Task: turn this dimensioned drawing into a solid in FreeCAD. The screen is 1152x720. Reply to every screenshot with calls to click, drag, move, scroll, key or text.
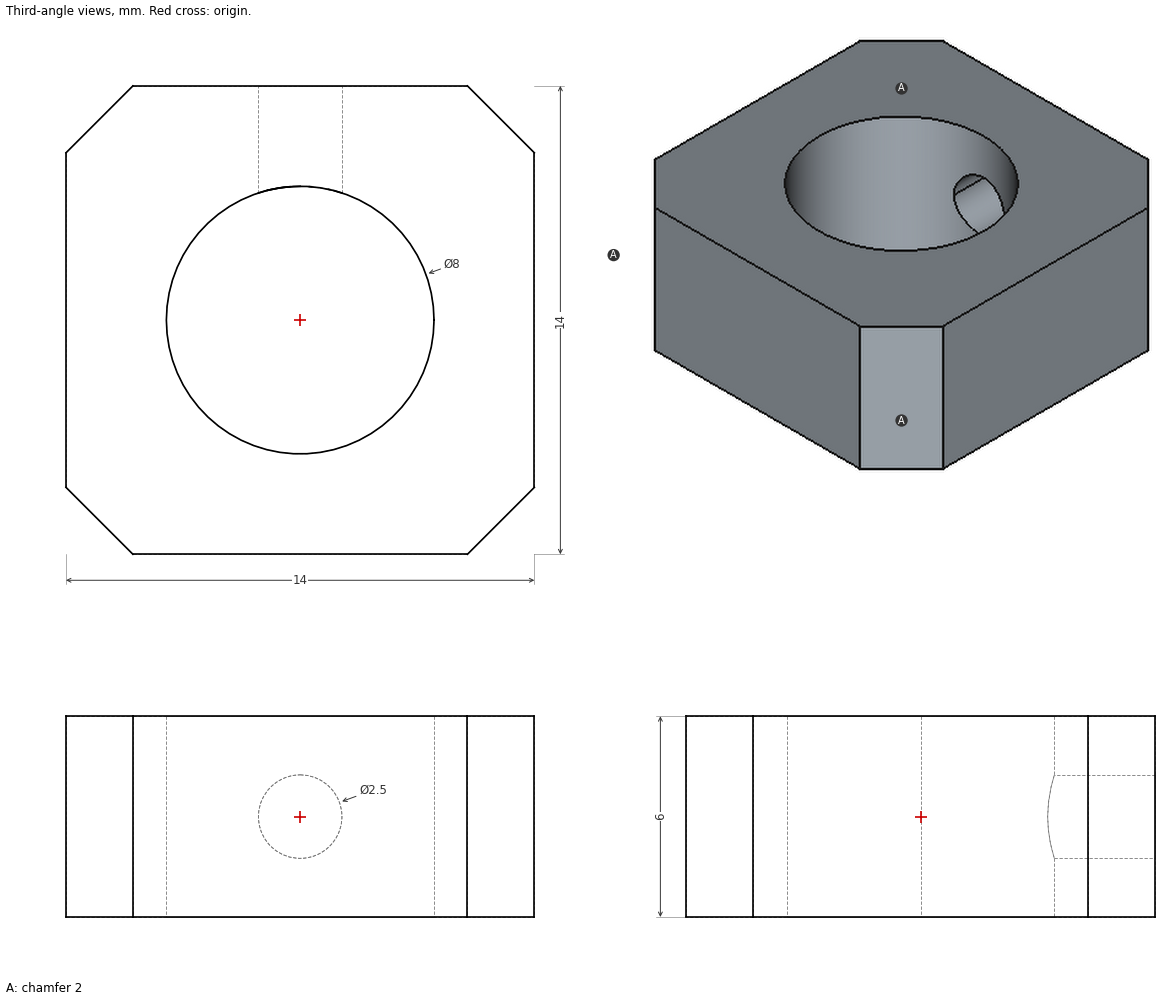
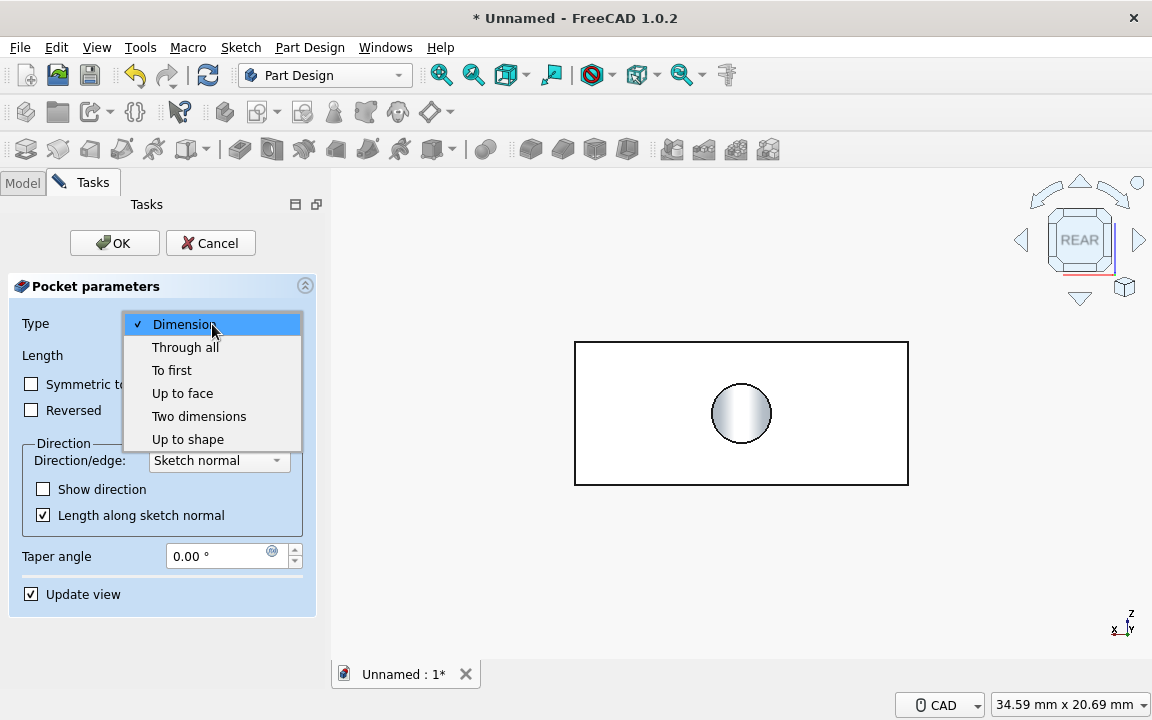
click(212, 370)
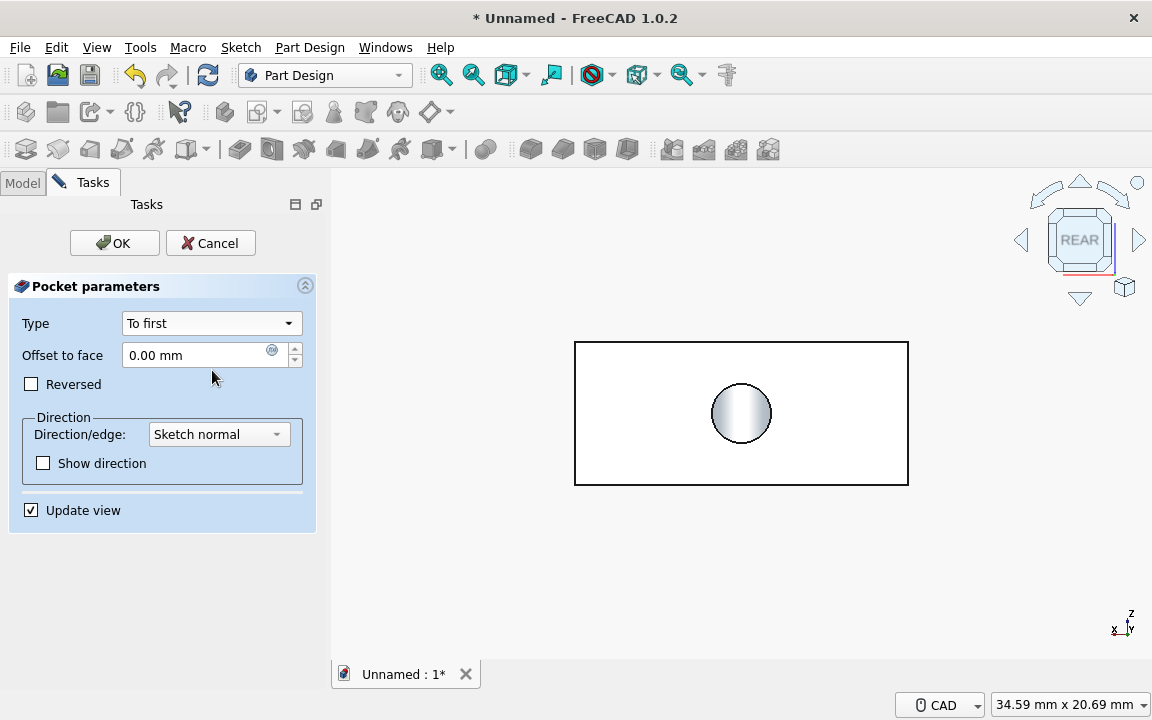
click(115, 243)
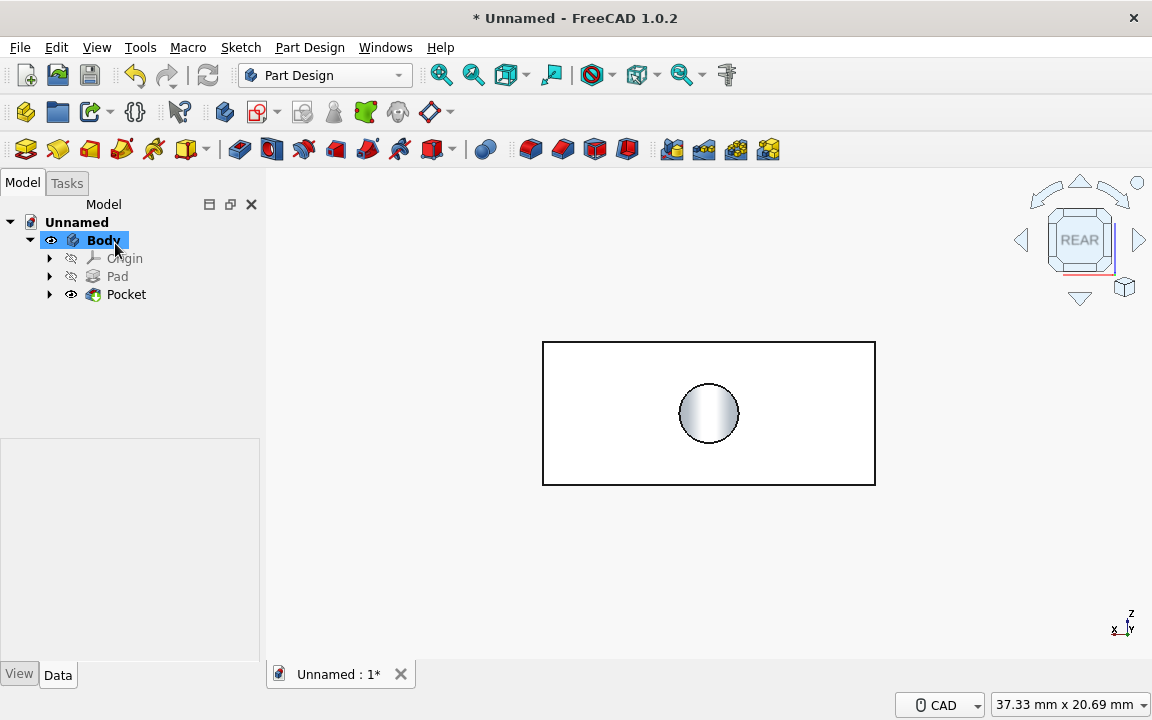
click(442, 76)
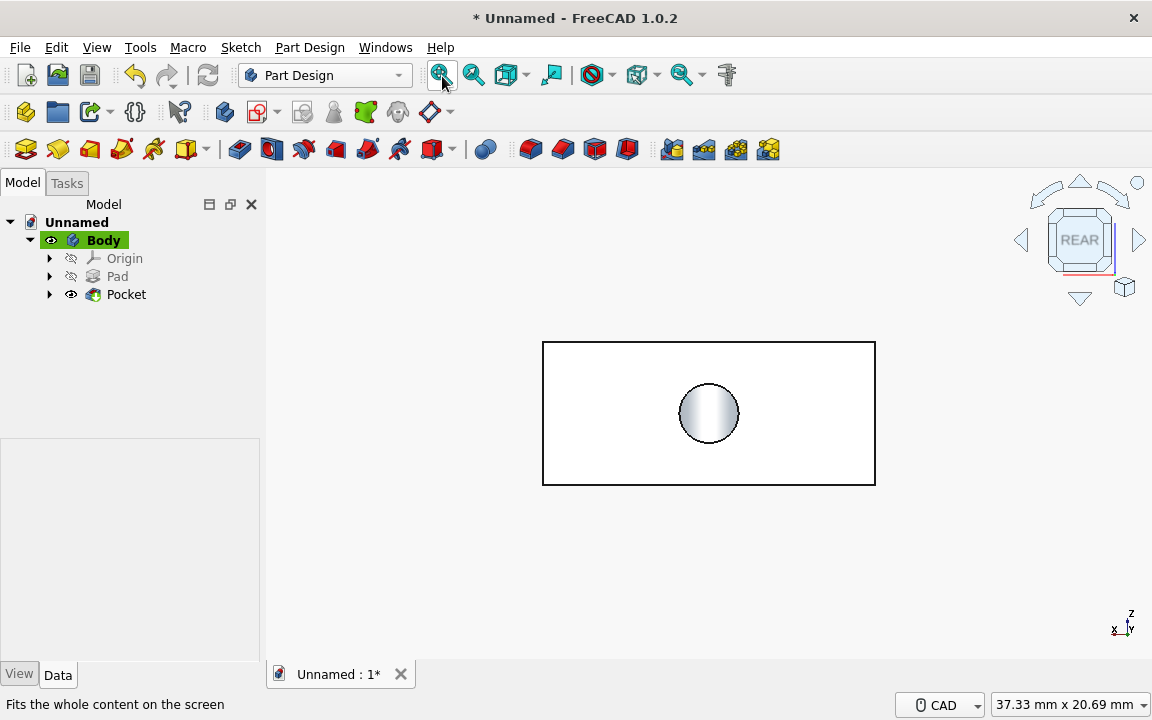
click(875, 412)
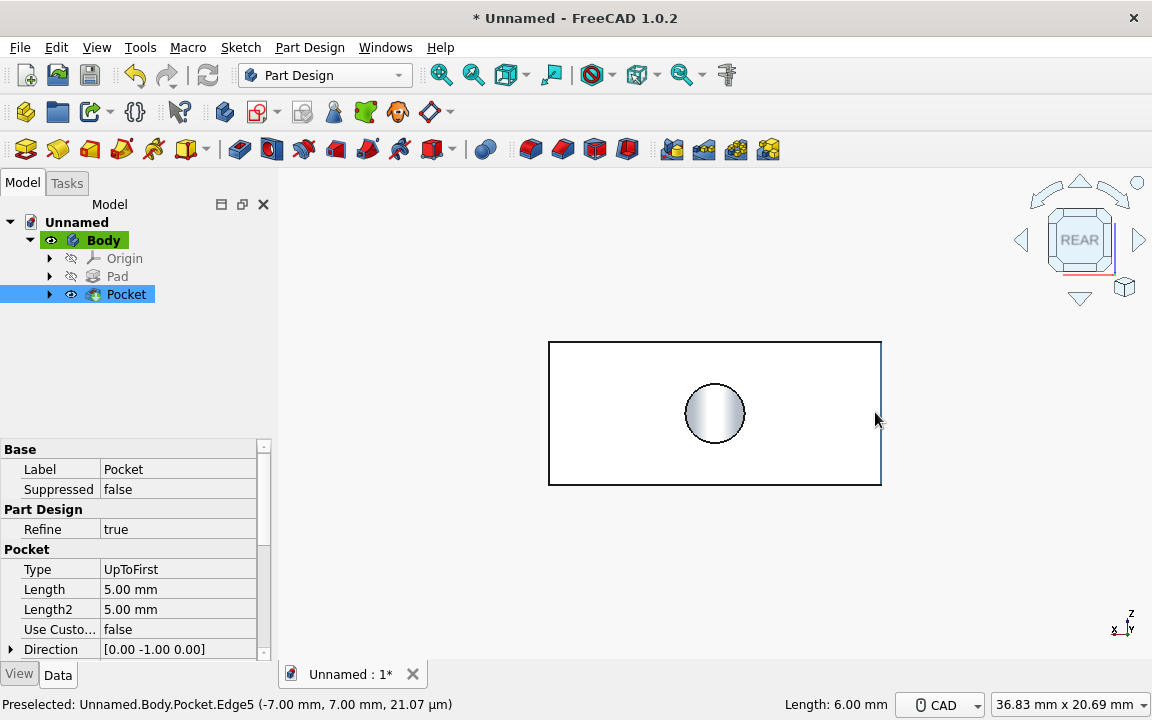
key(0)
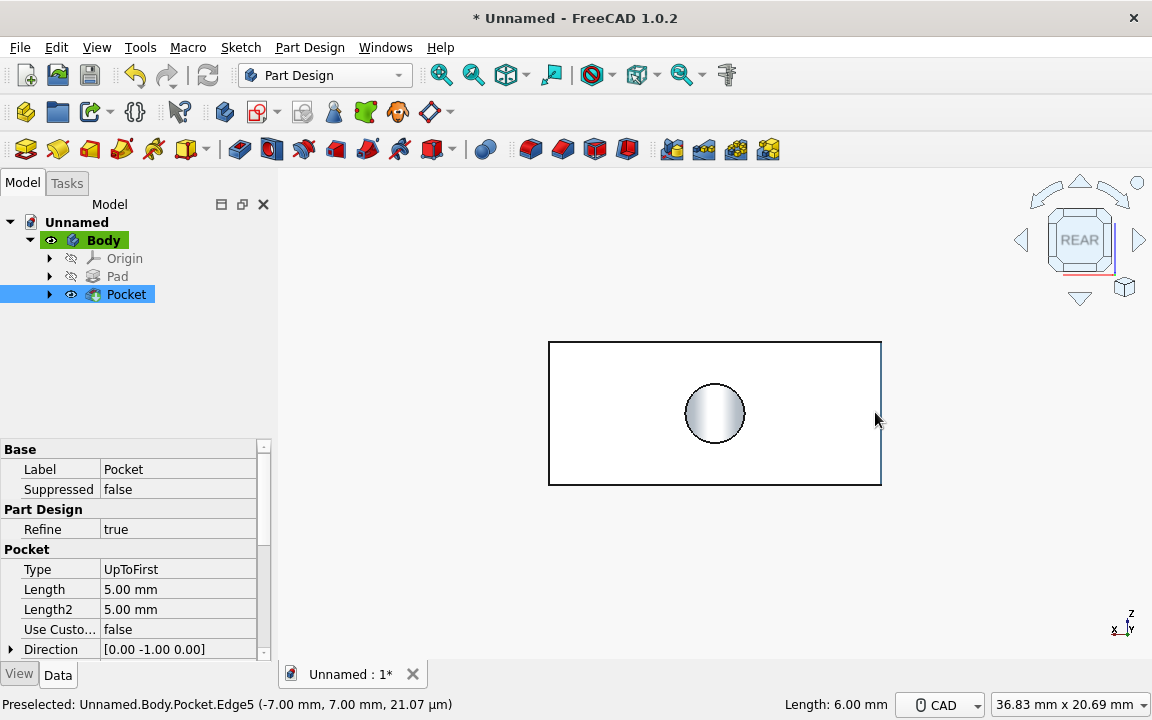
click(715, 548, ctrl)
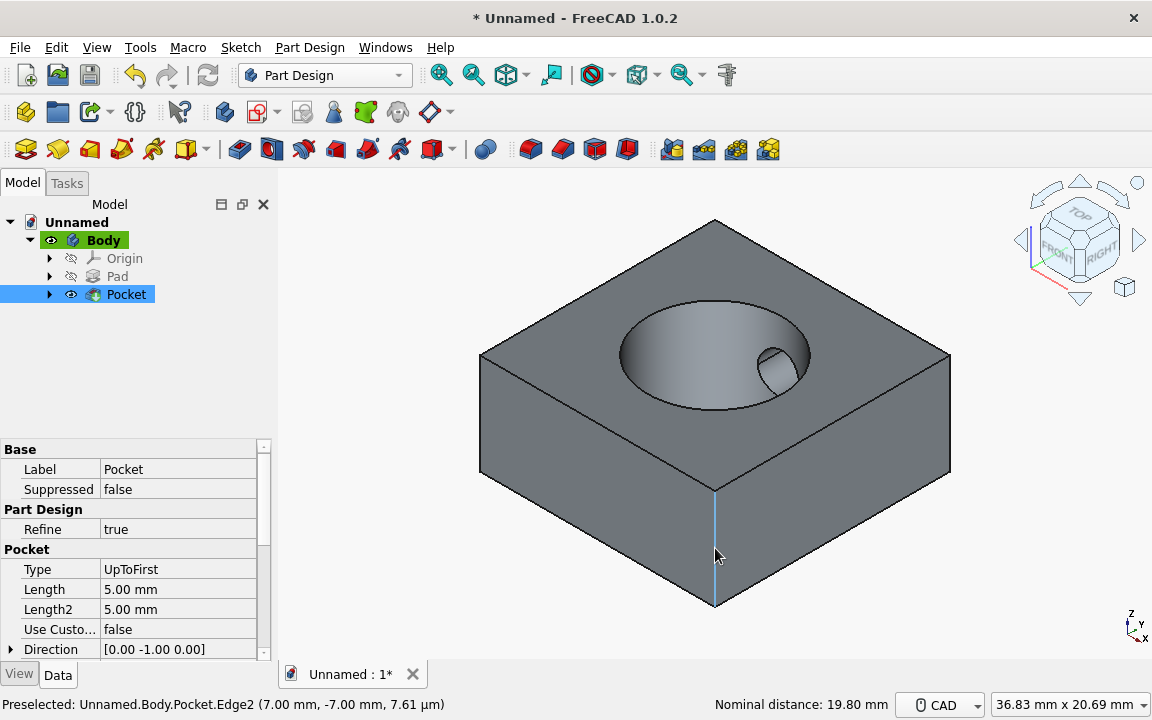
key(2)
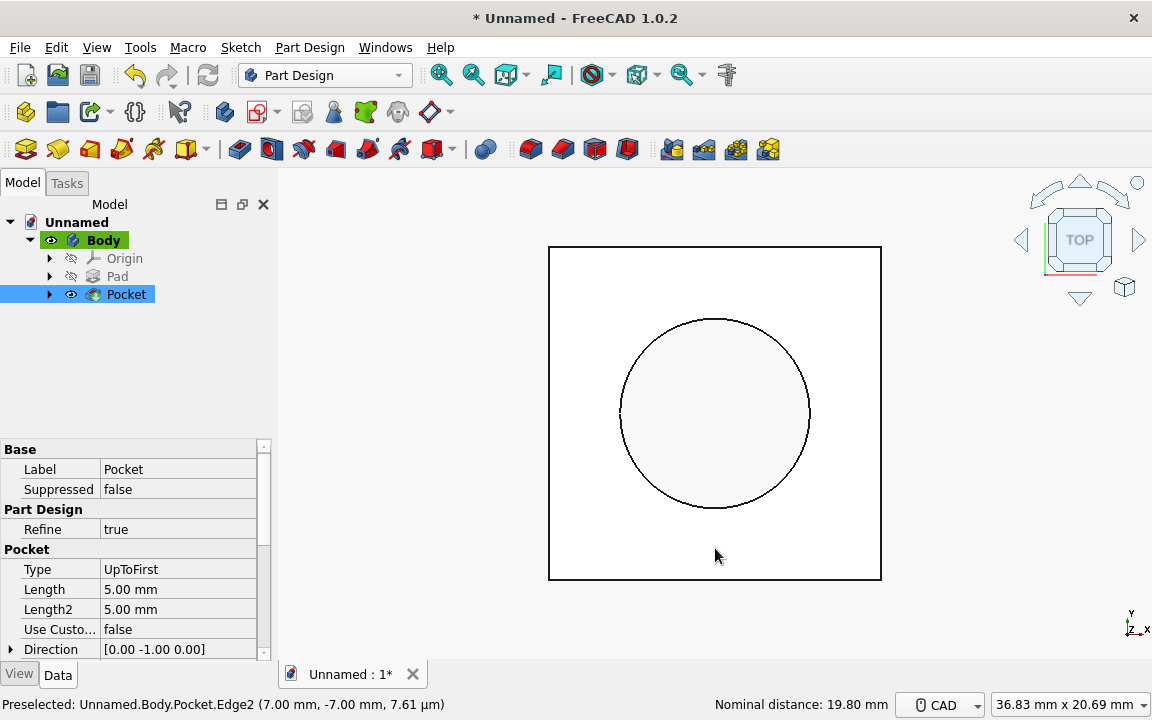
key(1)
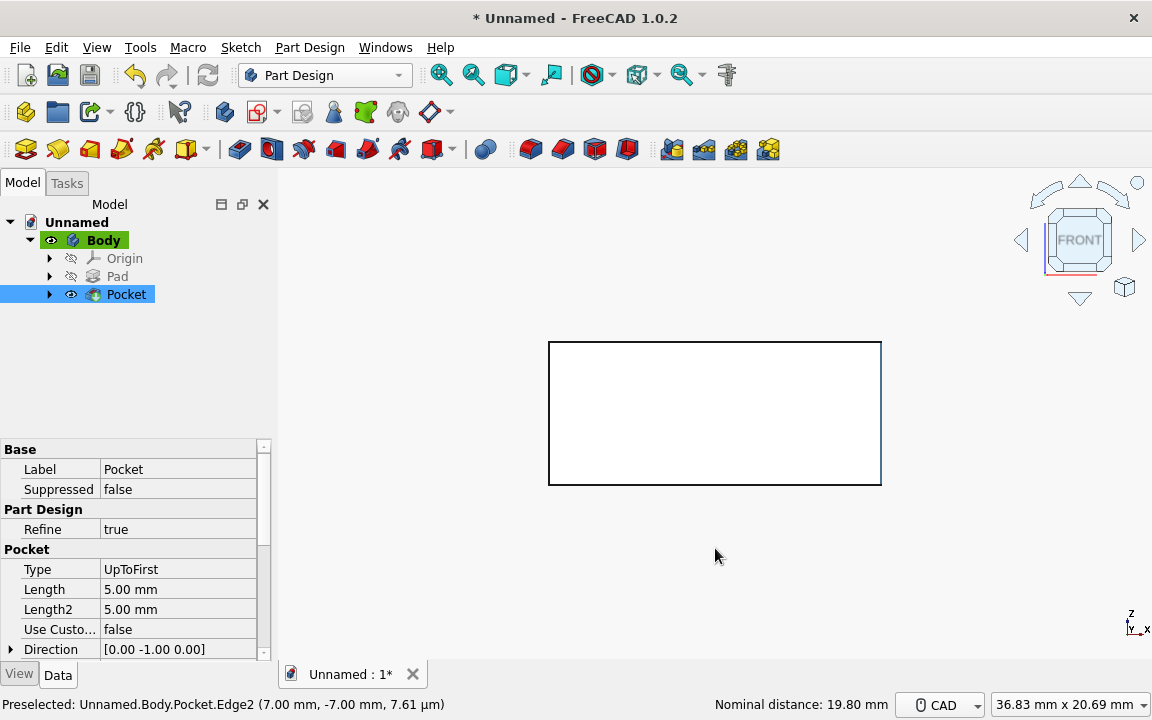
click(442, 76)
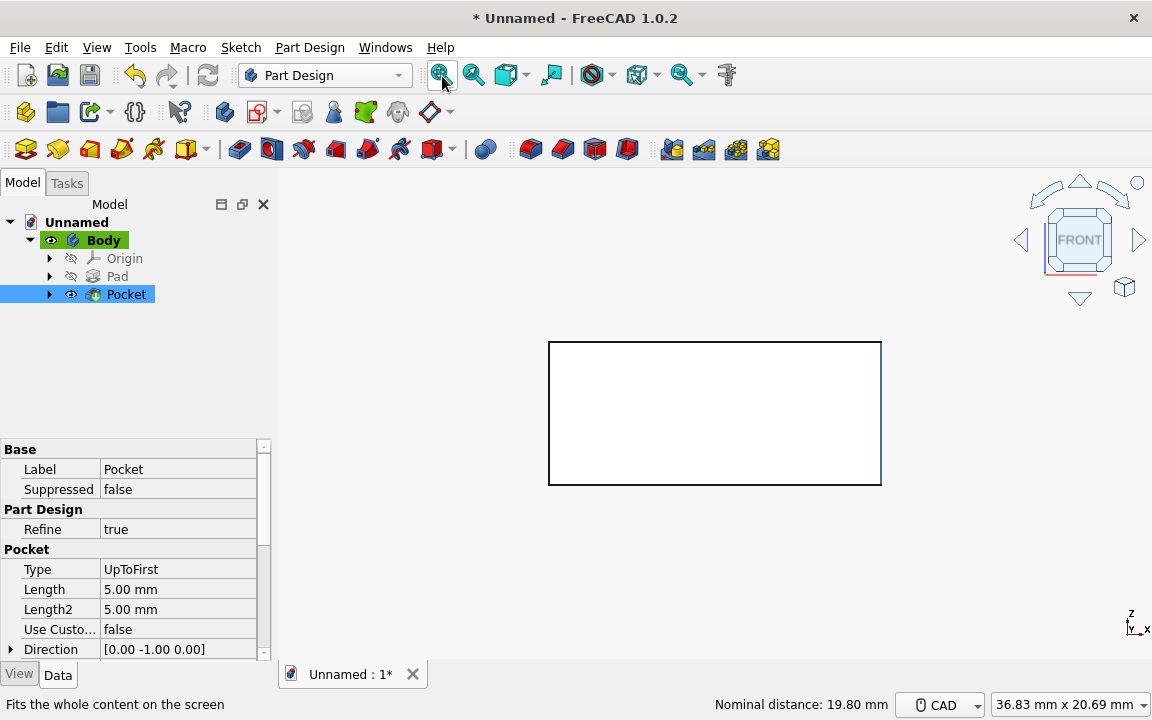
click(549, 413, ctrl)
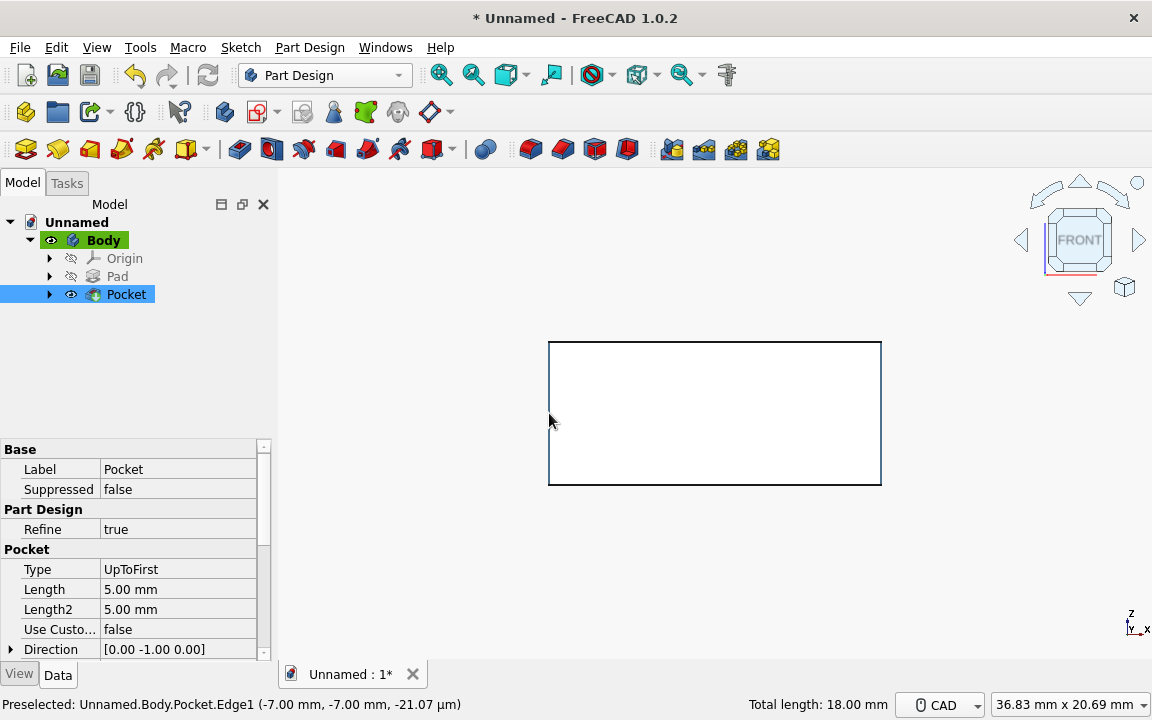
key(3)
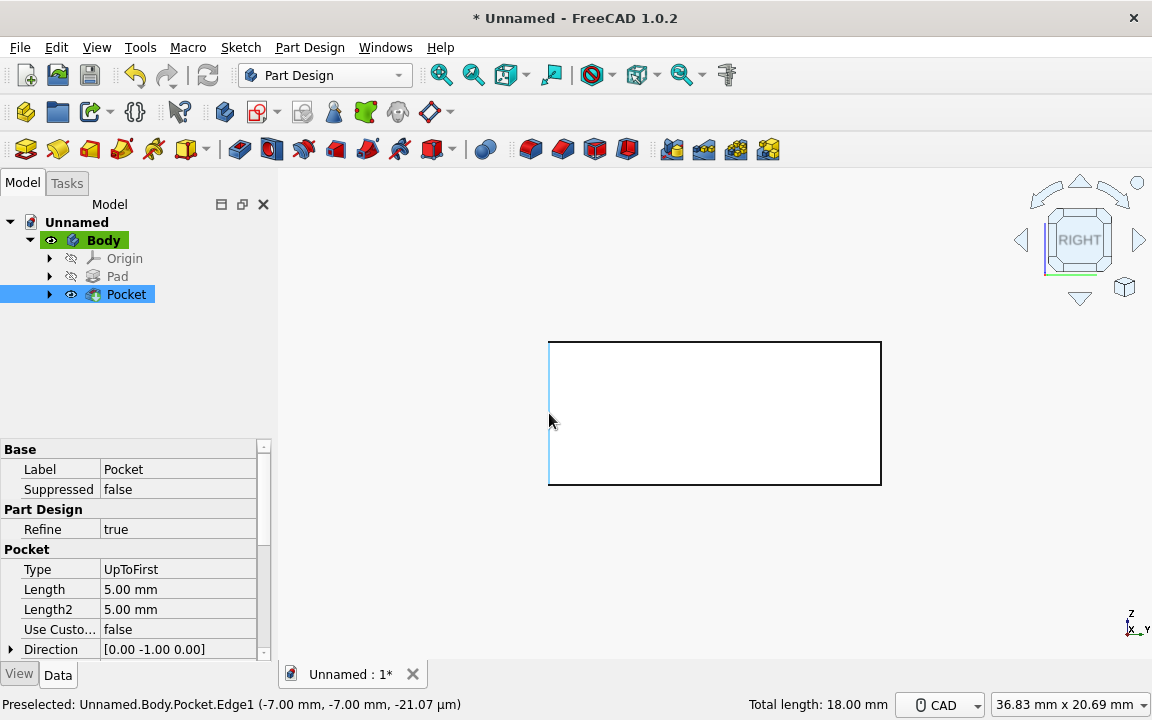
click(442, 76)